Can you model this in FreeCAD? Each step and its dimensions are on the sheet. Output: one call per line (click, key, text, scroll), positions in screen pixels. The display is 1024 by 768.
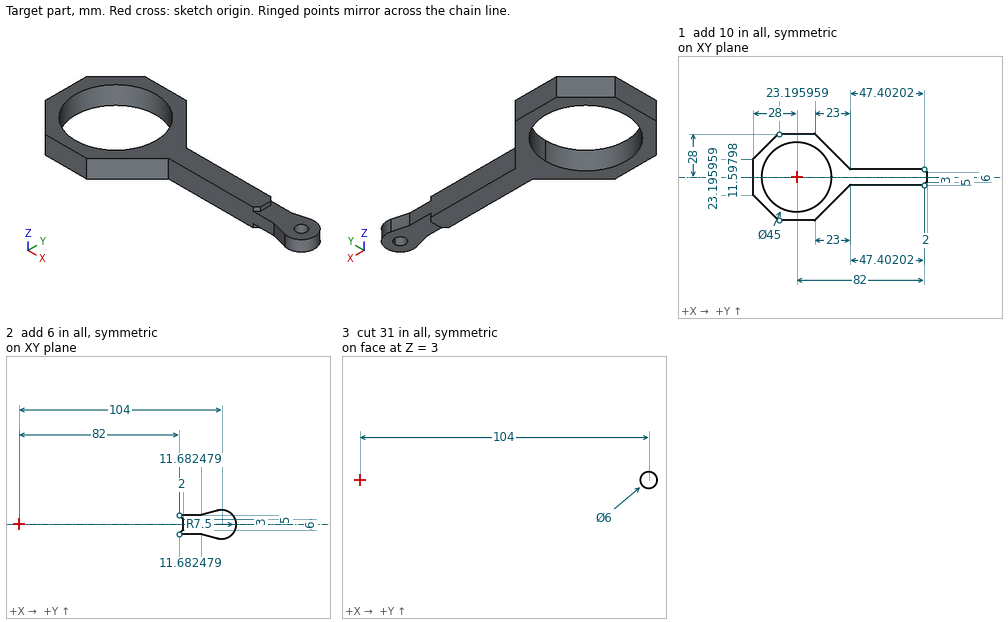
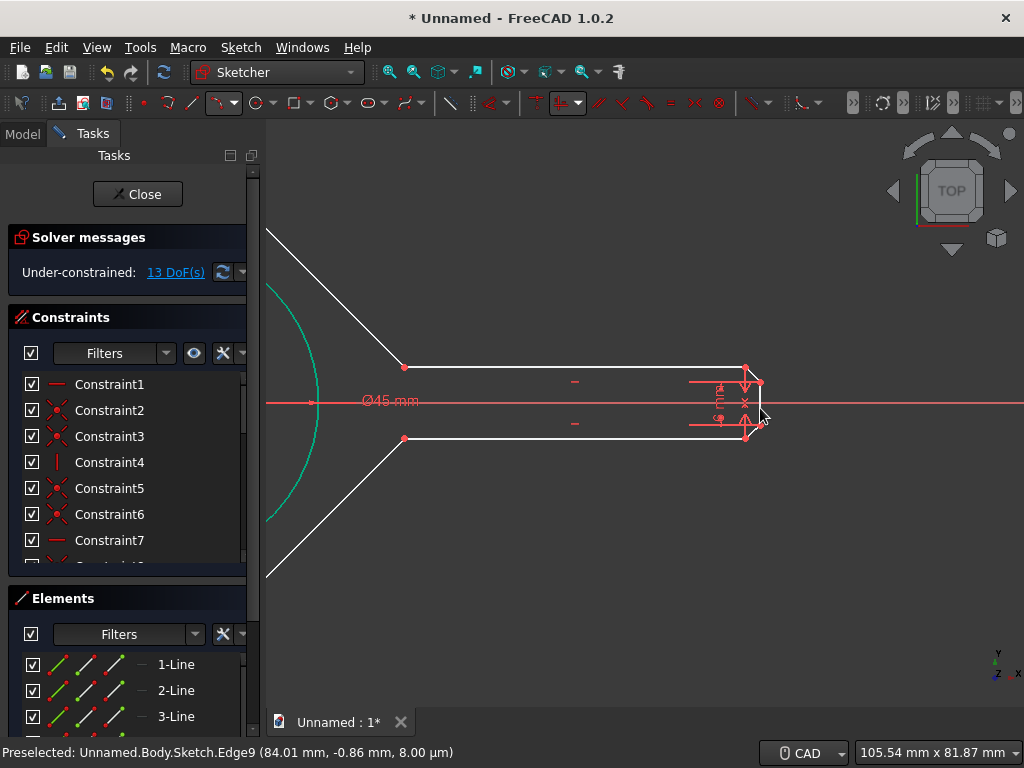
click(405, 438)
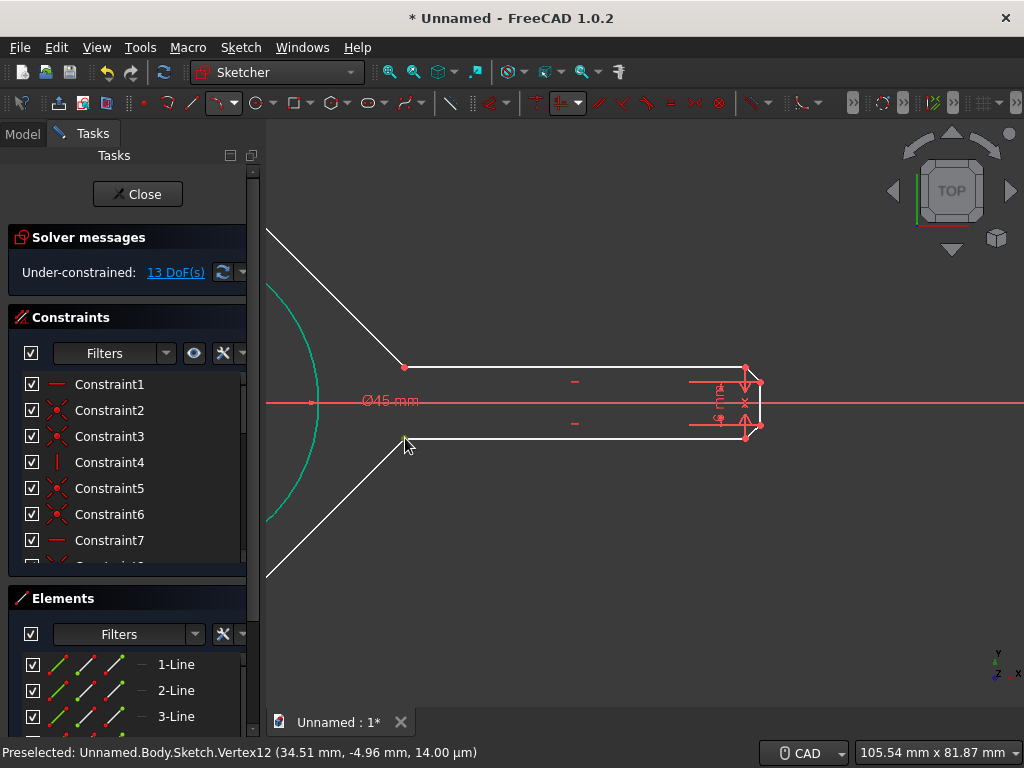
key(i)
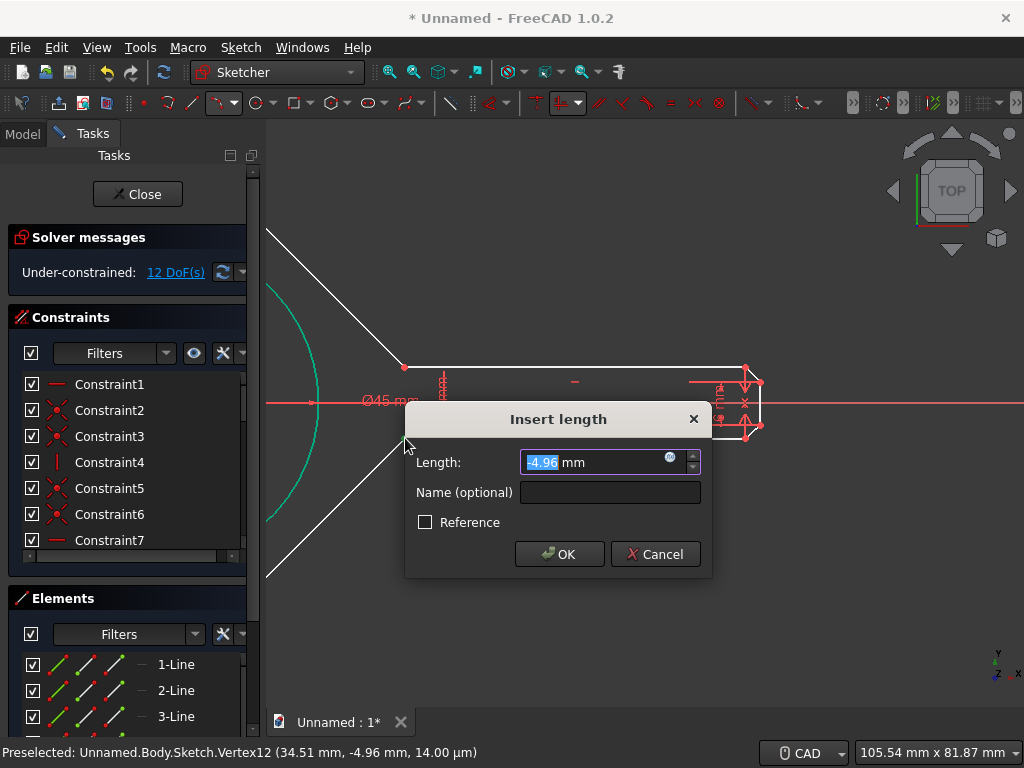
text(-5)
key(Return)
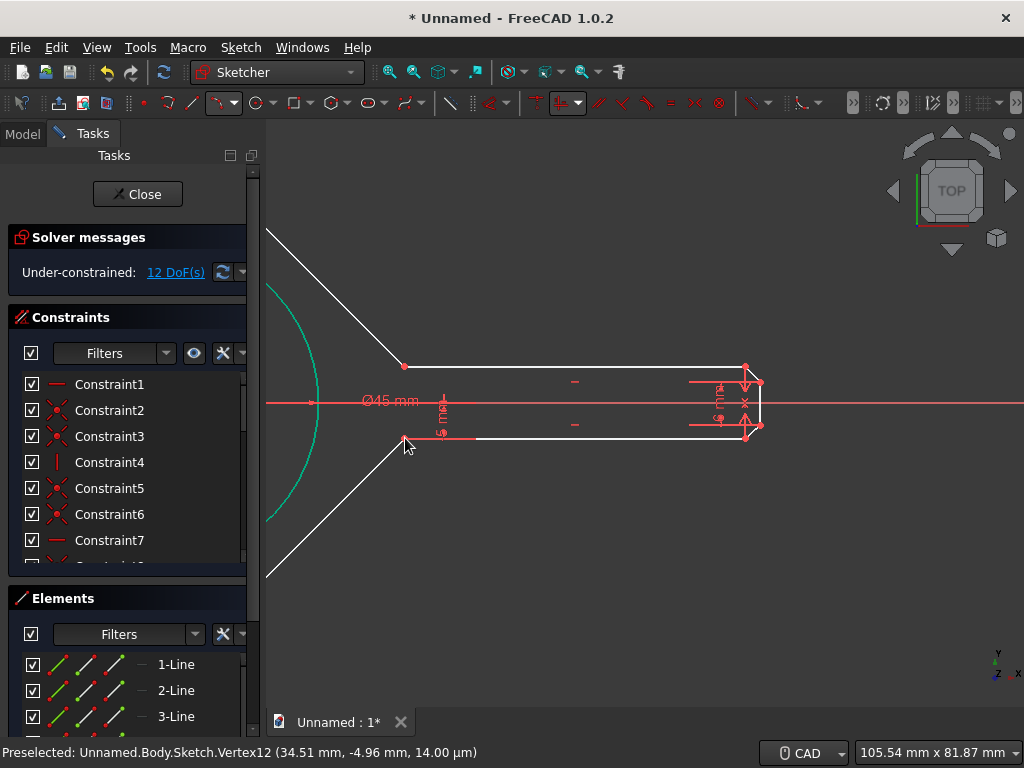
scroll(760, 425, up, 4)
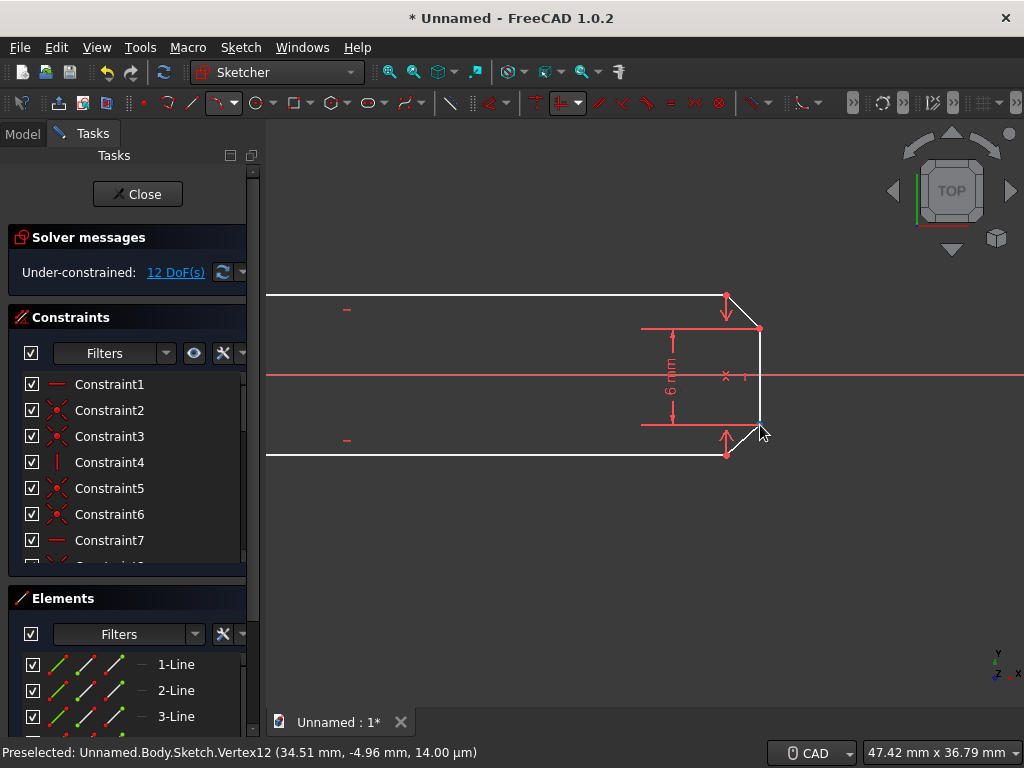
click(760, 425)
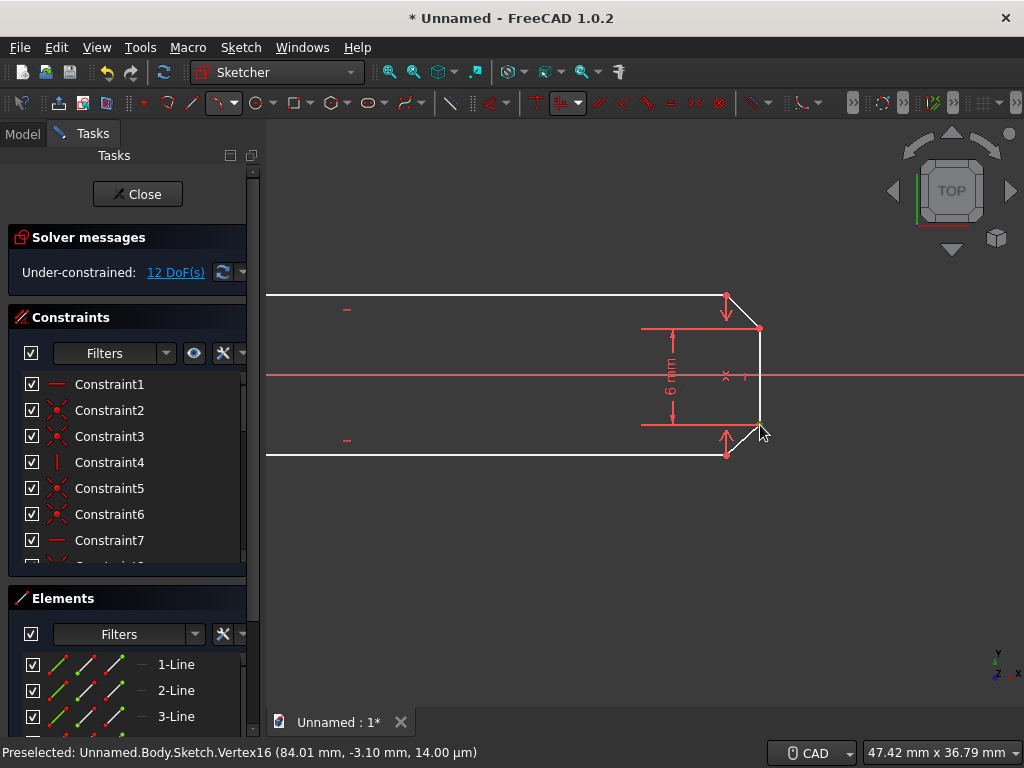
key(i)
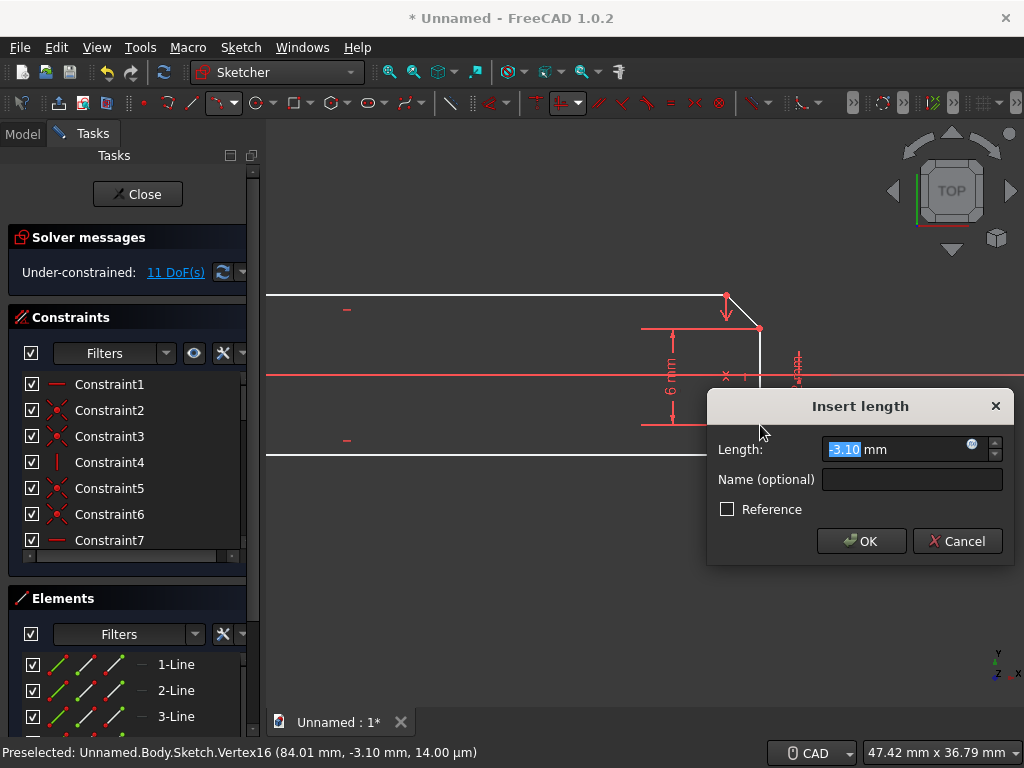
text(-3)
key(Return)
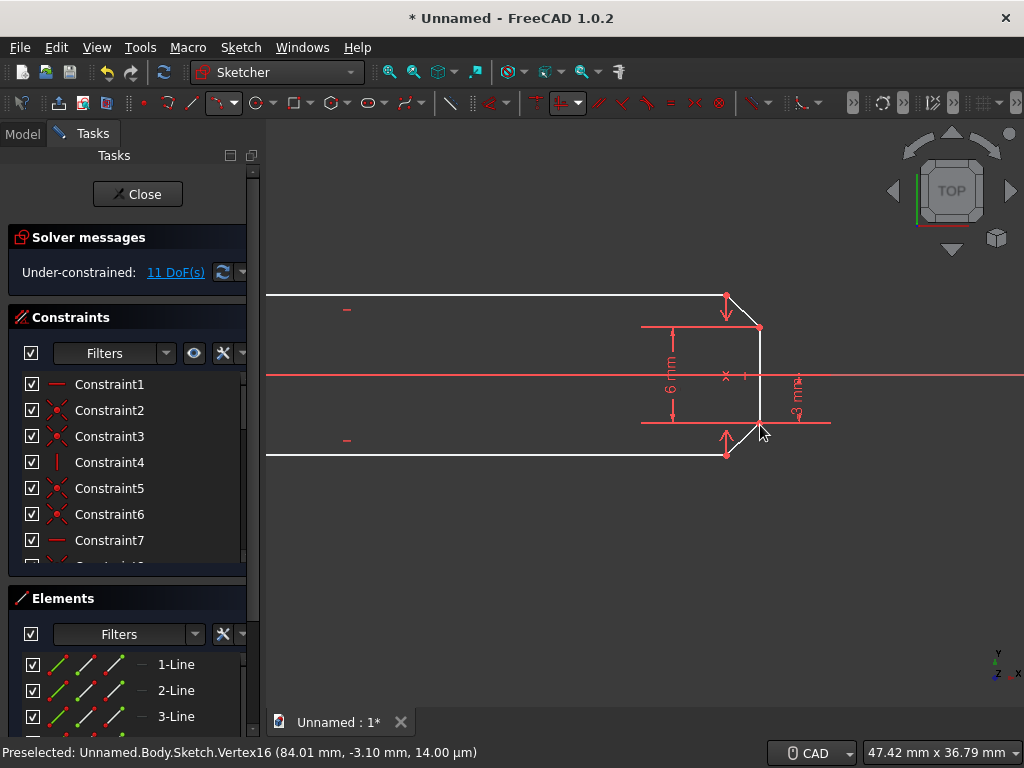
scroll(736, 445, up, 2)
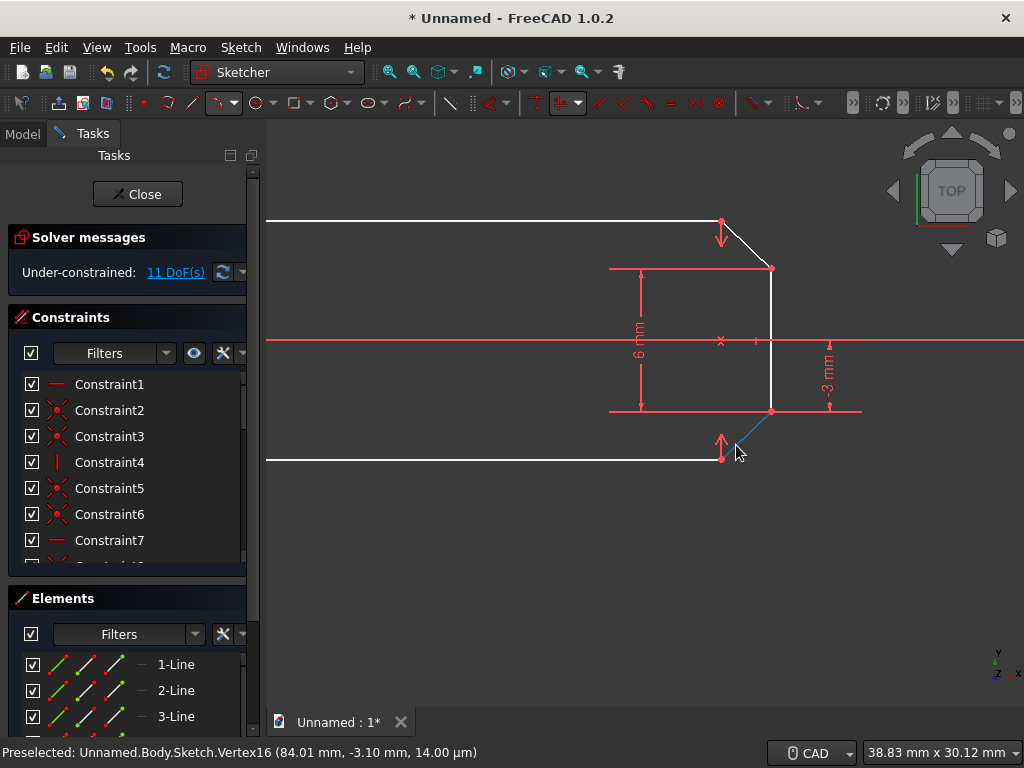
click(736, 445)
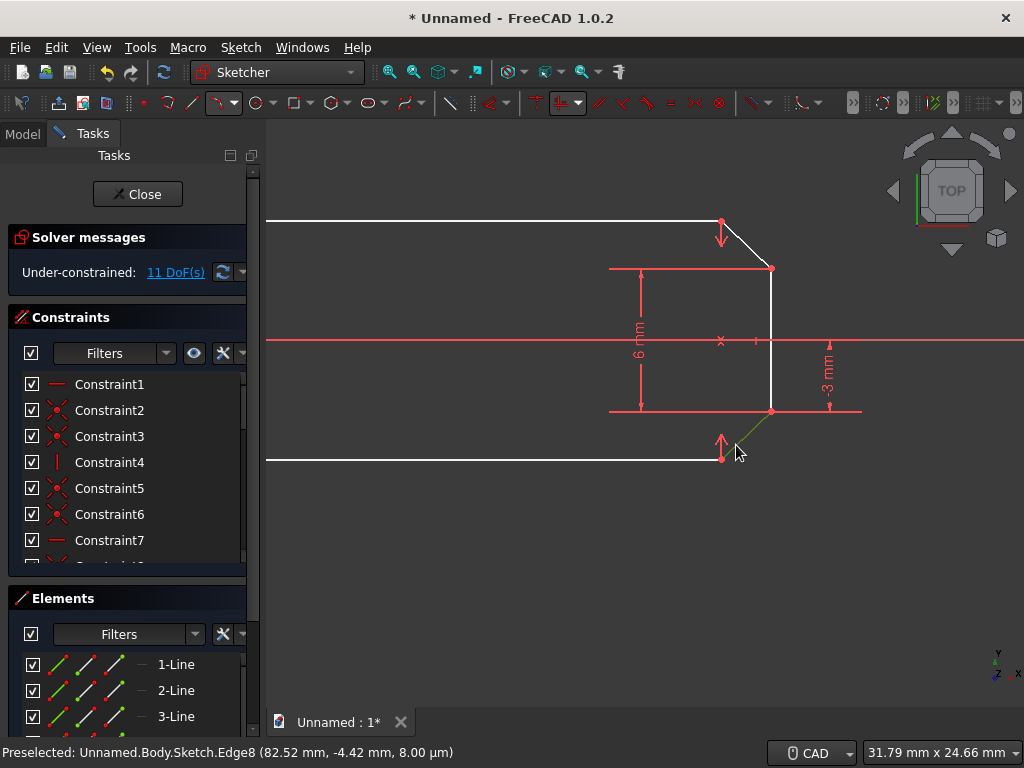
click(508, 104)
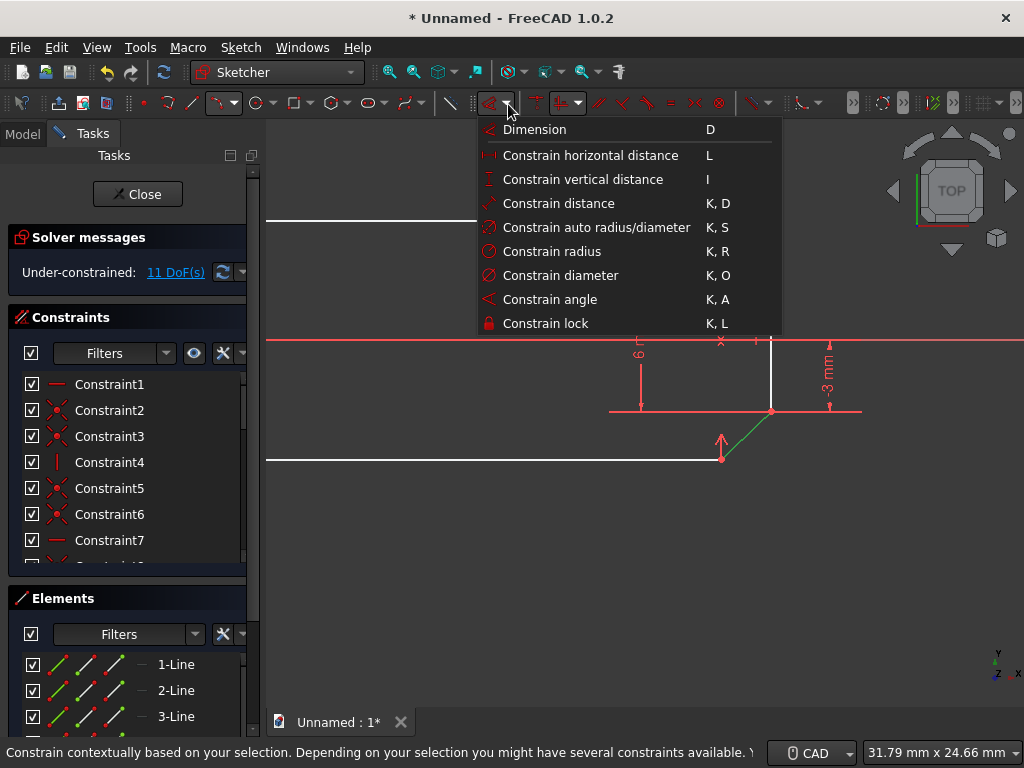
click(630, 155)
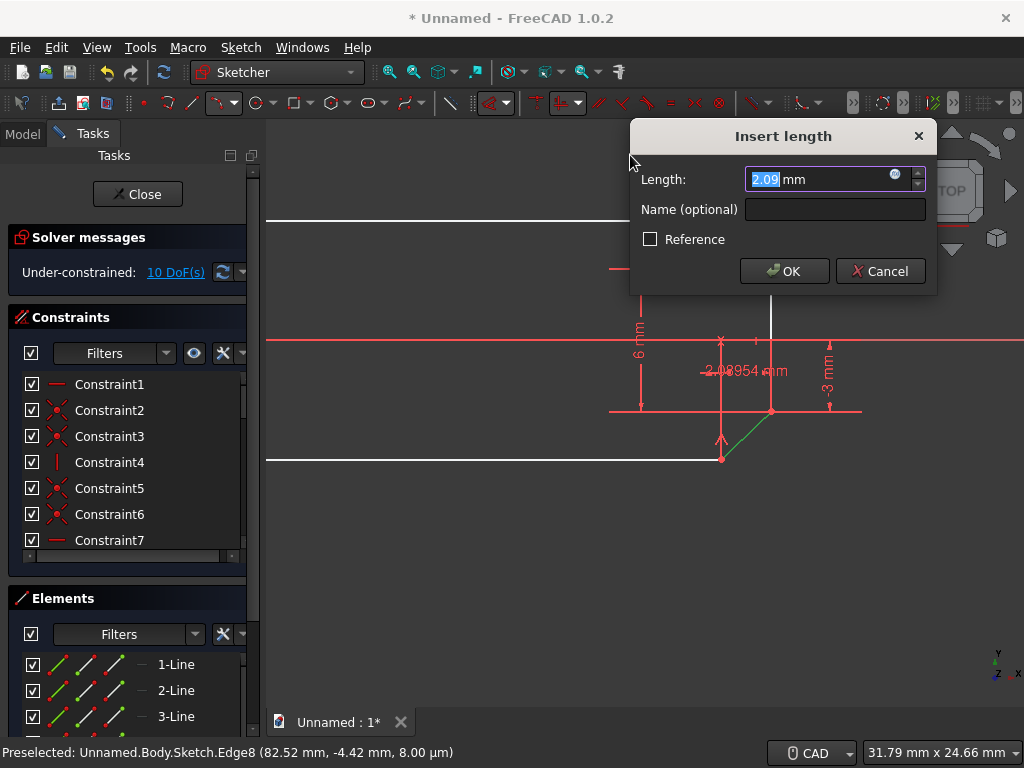
text(2)
key(Return)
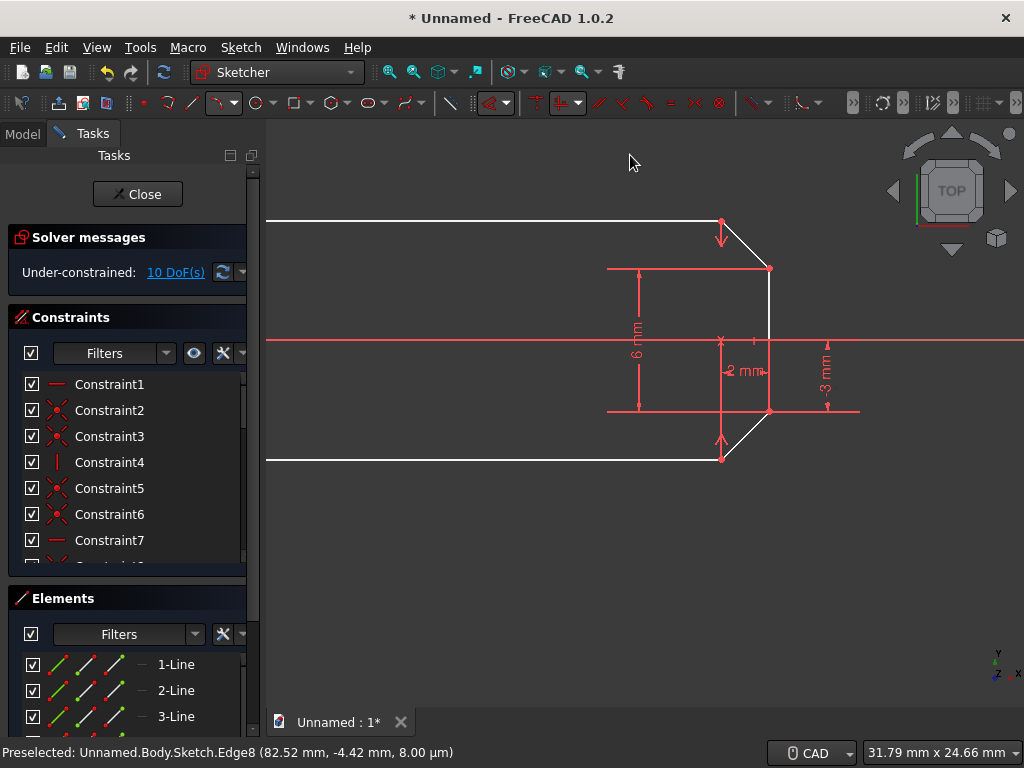
scroll(755, 424, down, 10)